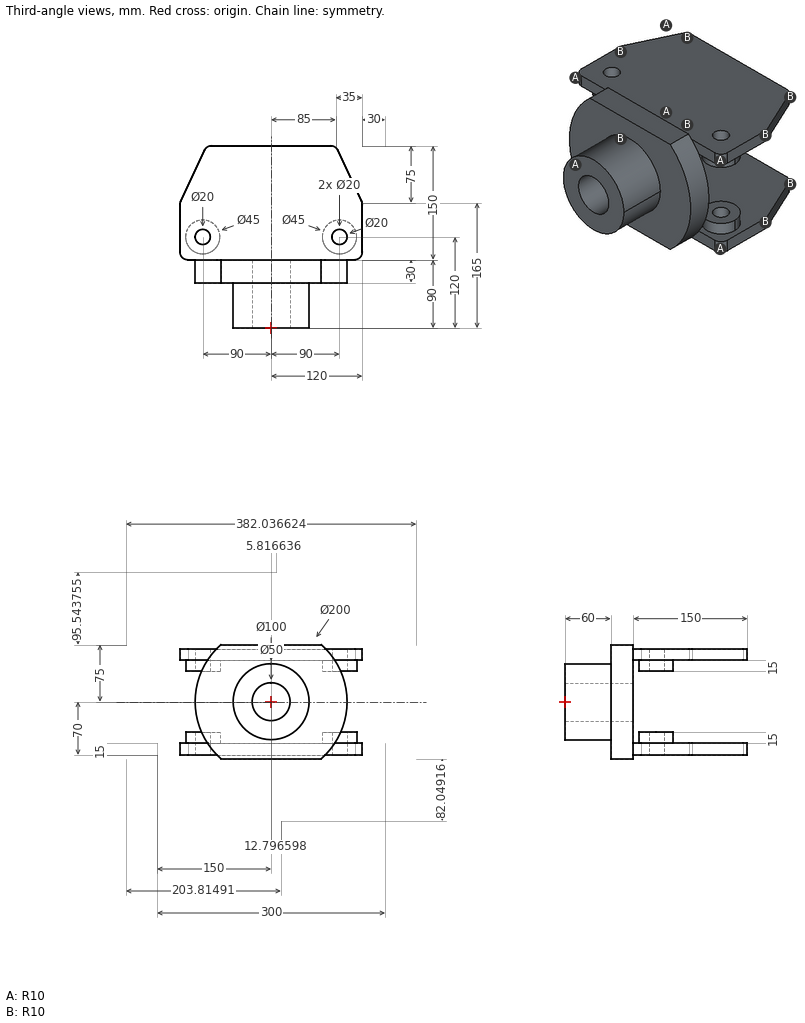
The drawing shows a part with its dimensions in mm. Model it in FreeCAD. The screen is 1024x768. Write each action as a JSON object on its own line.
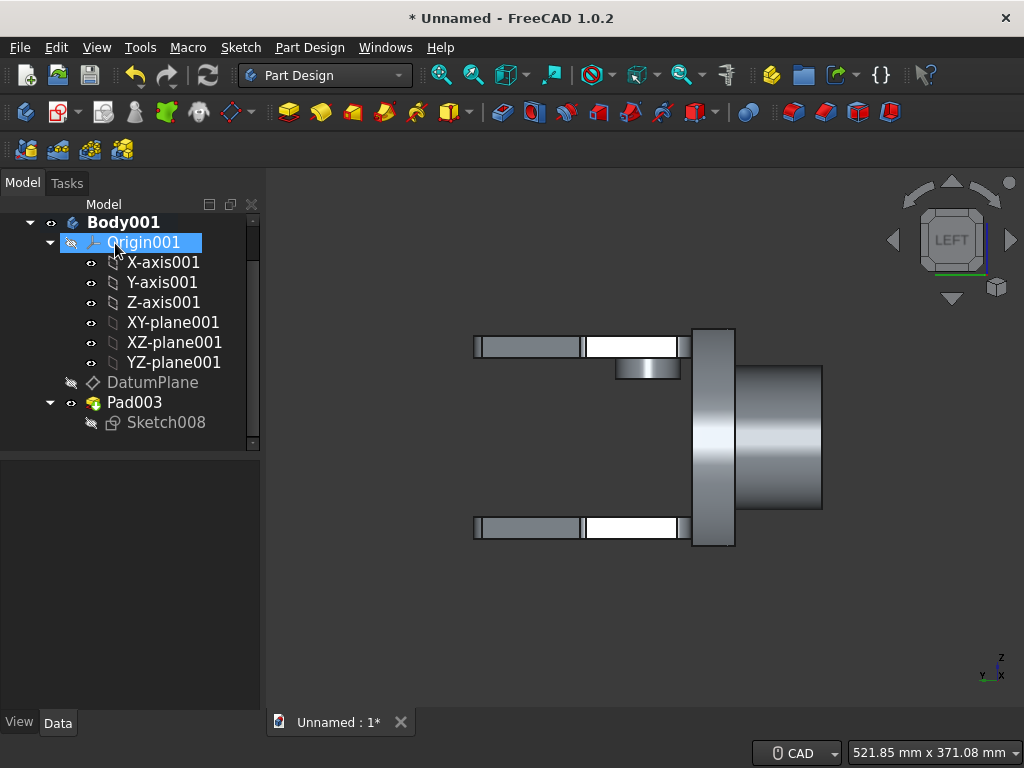
{"action": "left_click", "coordinate": [442, 76]}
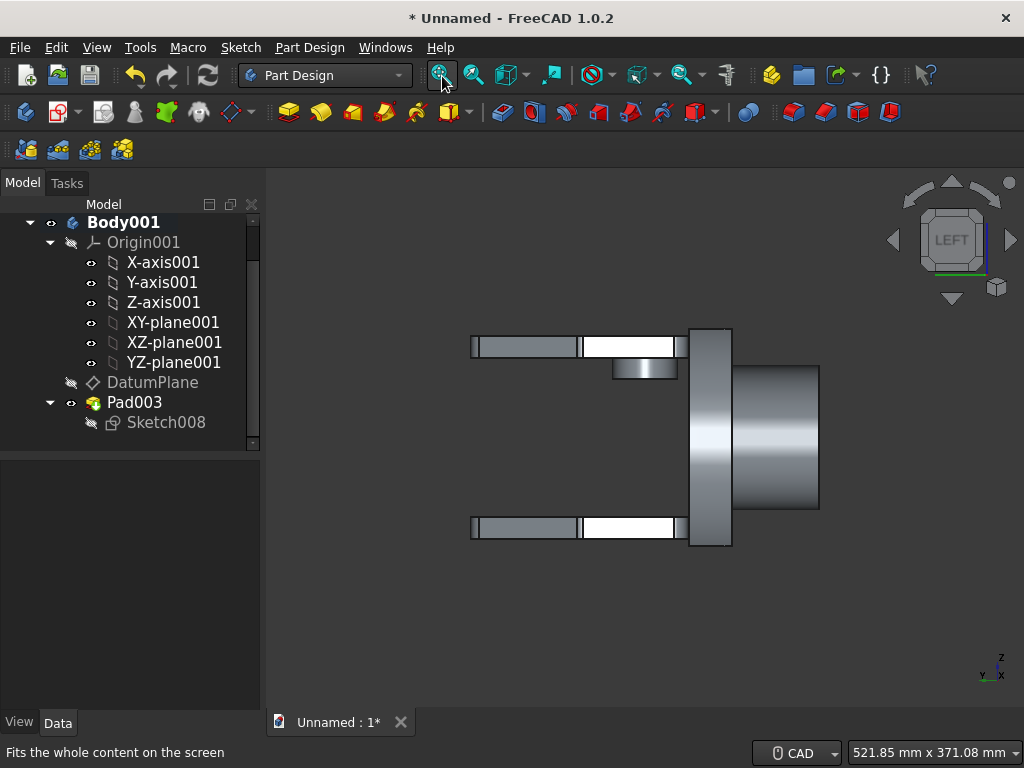
{"action": "left_click", "coordinate": [26, 112]}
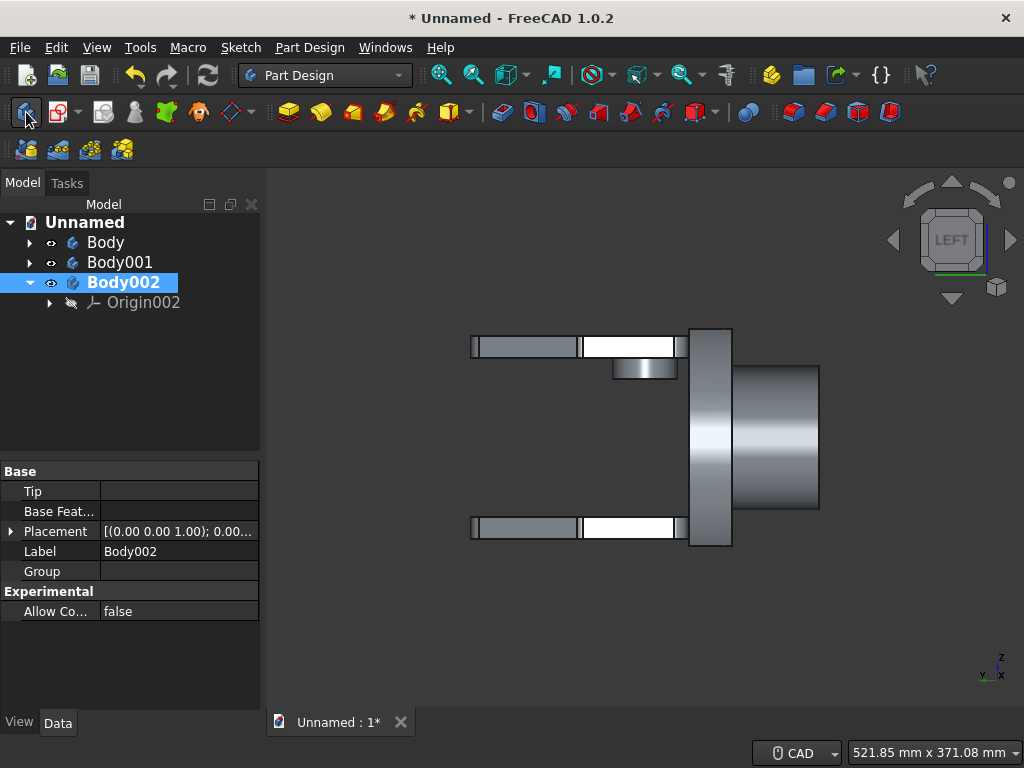
{"action": "left_click", "coordinate": [50, 303]}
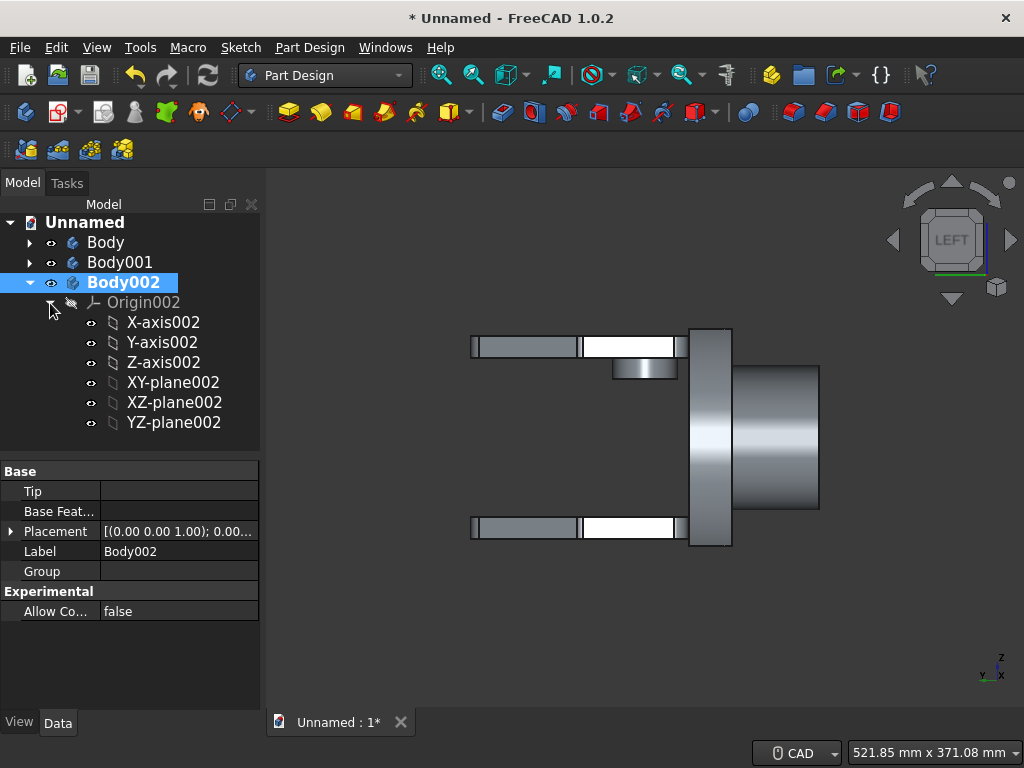
{"action": "left_click", "coordinate": [136, 383]}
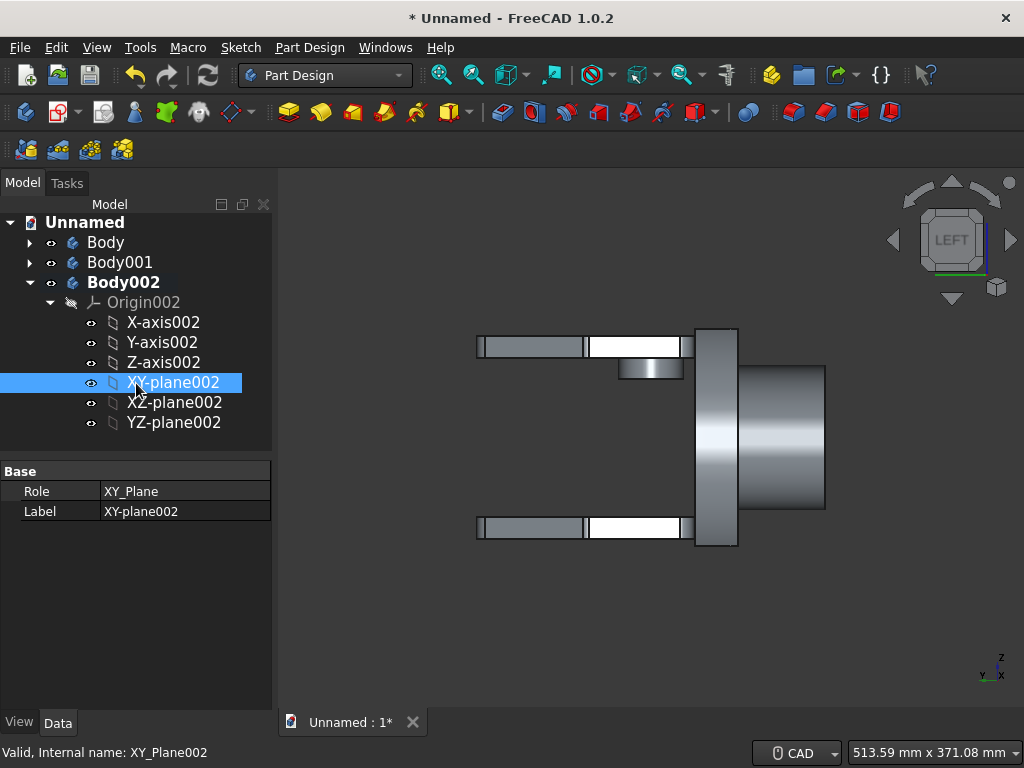
{"action": "left_click", "coordinate": [232, 112]}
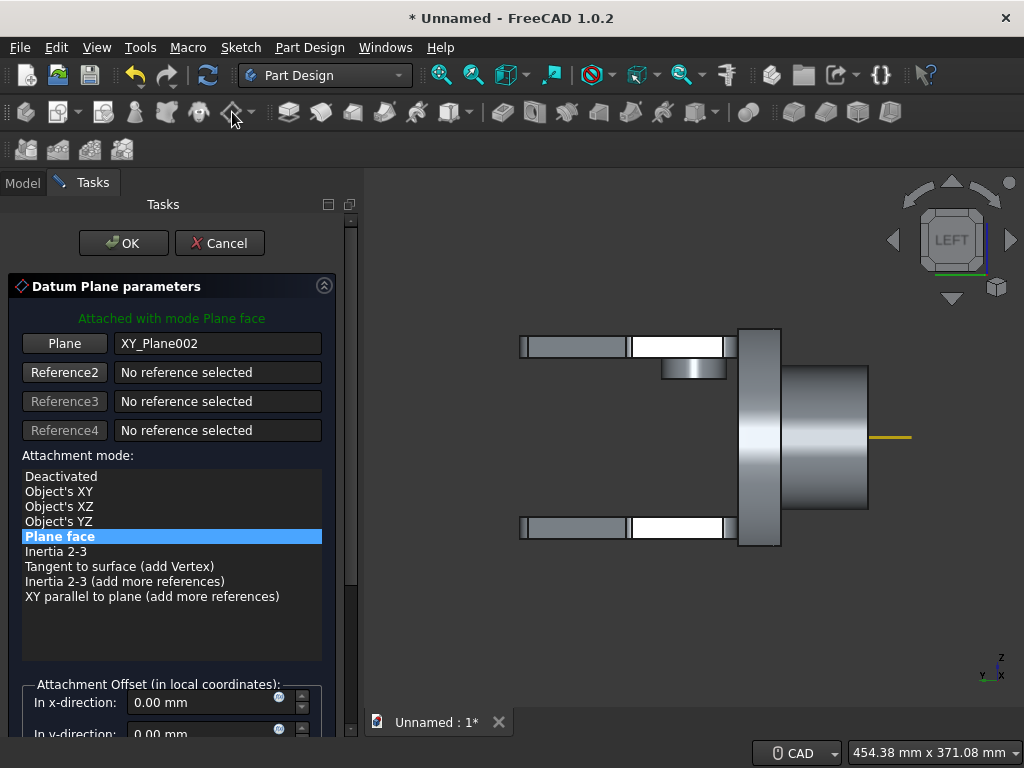
{"action": "scroll", "coordinate": [351, 475], "scroll_direction": "down", "scroll_amount": 2}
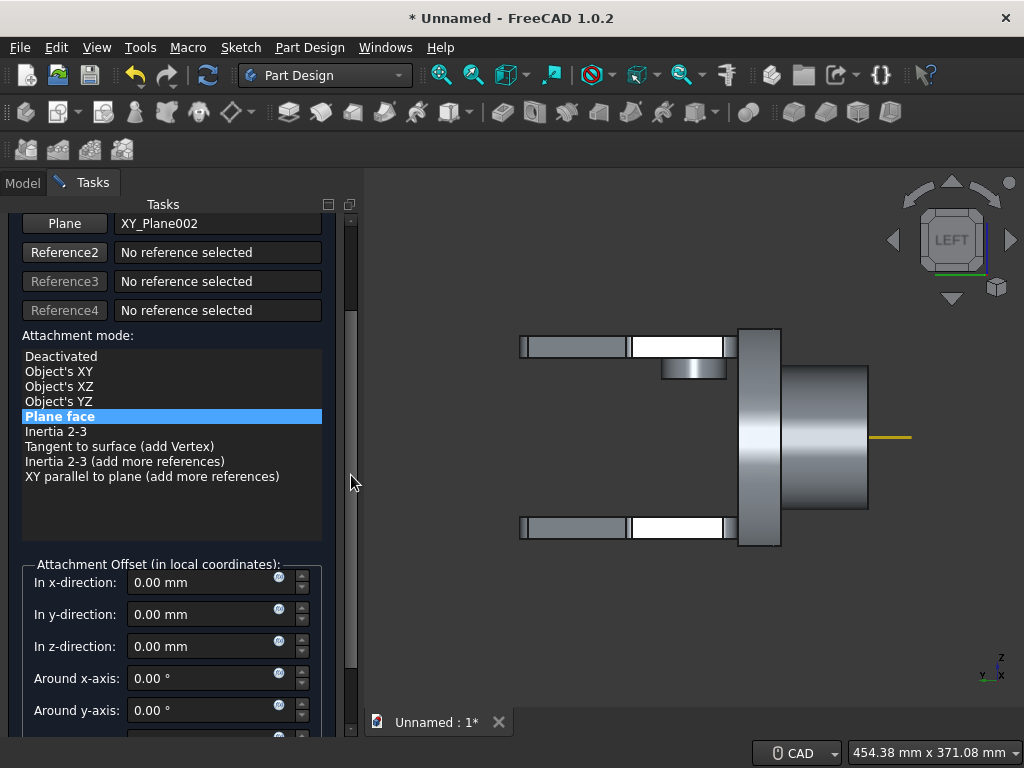
{"action": "triple_click", "coordinate": [210, 646]}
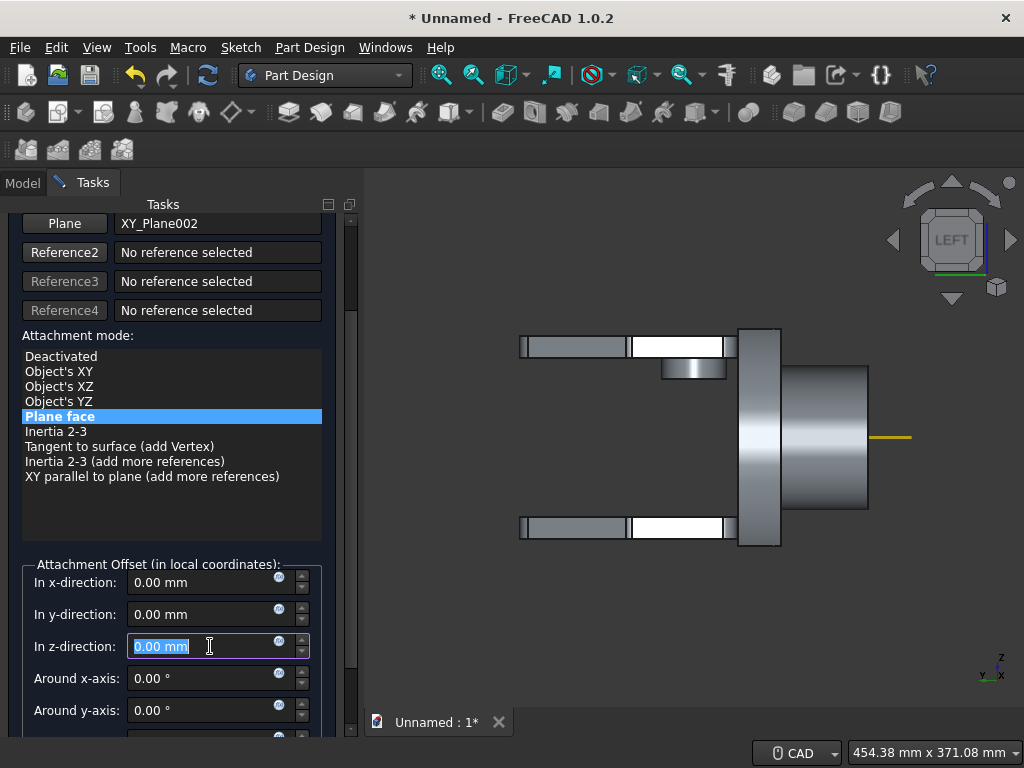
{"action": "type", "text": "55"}
{"action": "key", "text": "Tab"}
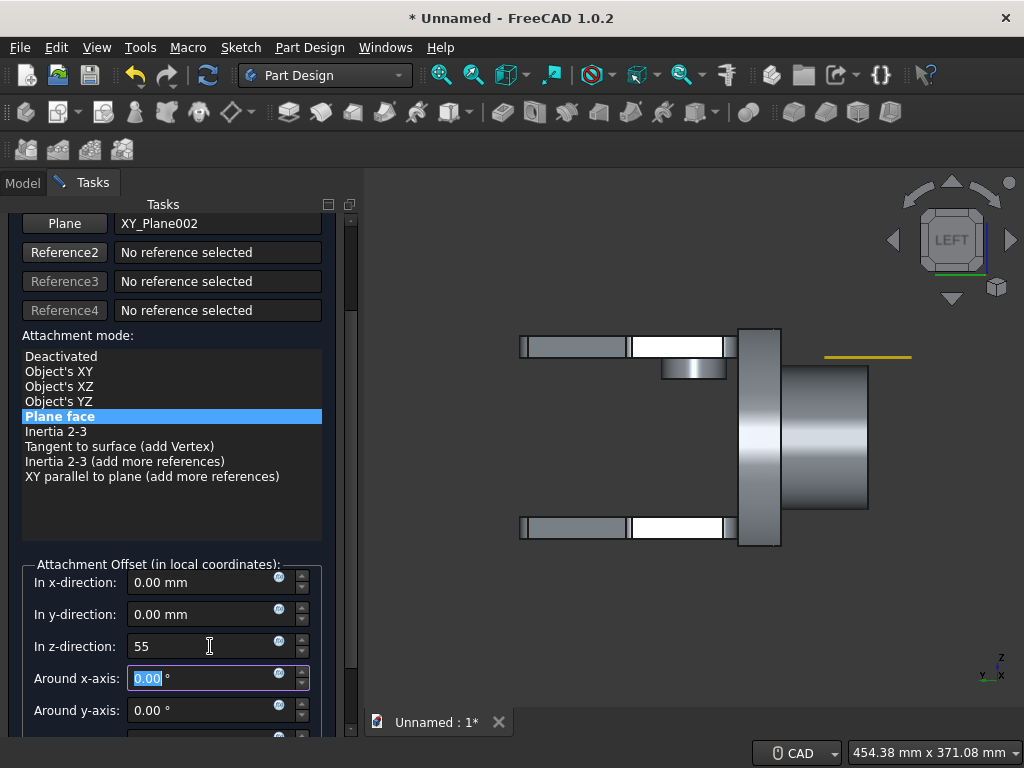
{"action": "scroll", "coordinate": [351, 475], "scroll_direction": "up", "scroll_amount": 3}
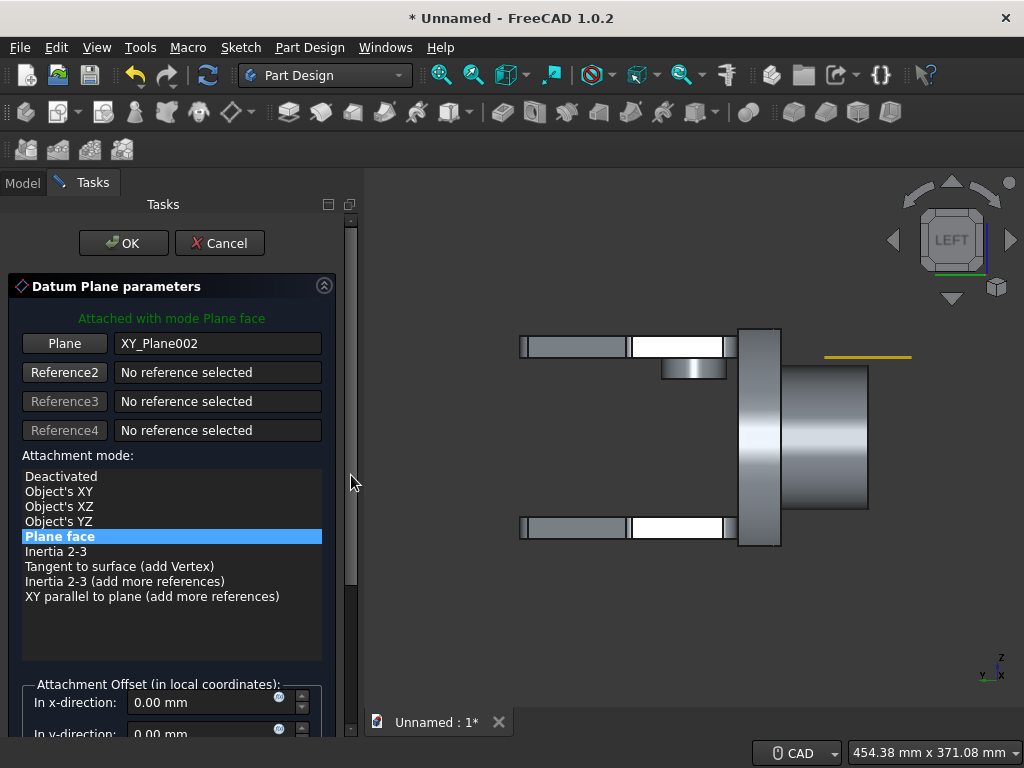
{"action": "left_click", "coordinate": [124, 243]}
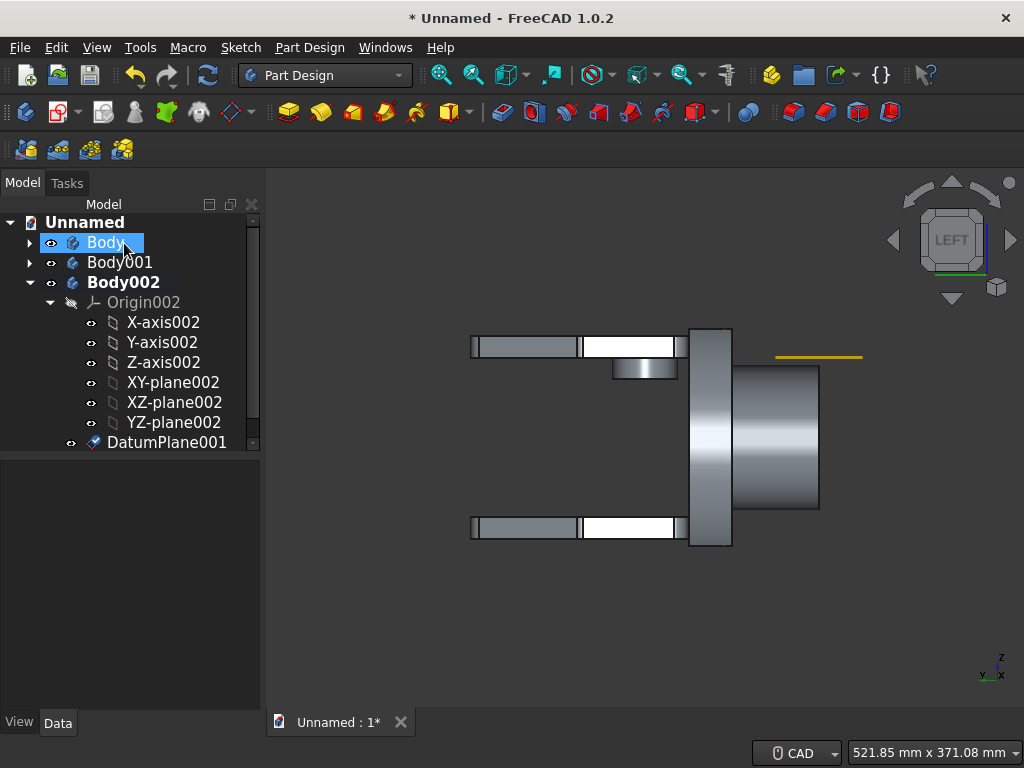
{"action": "left_click", "coordinate": [116, 443]}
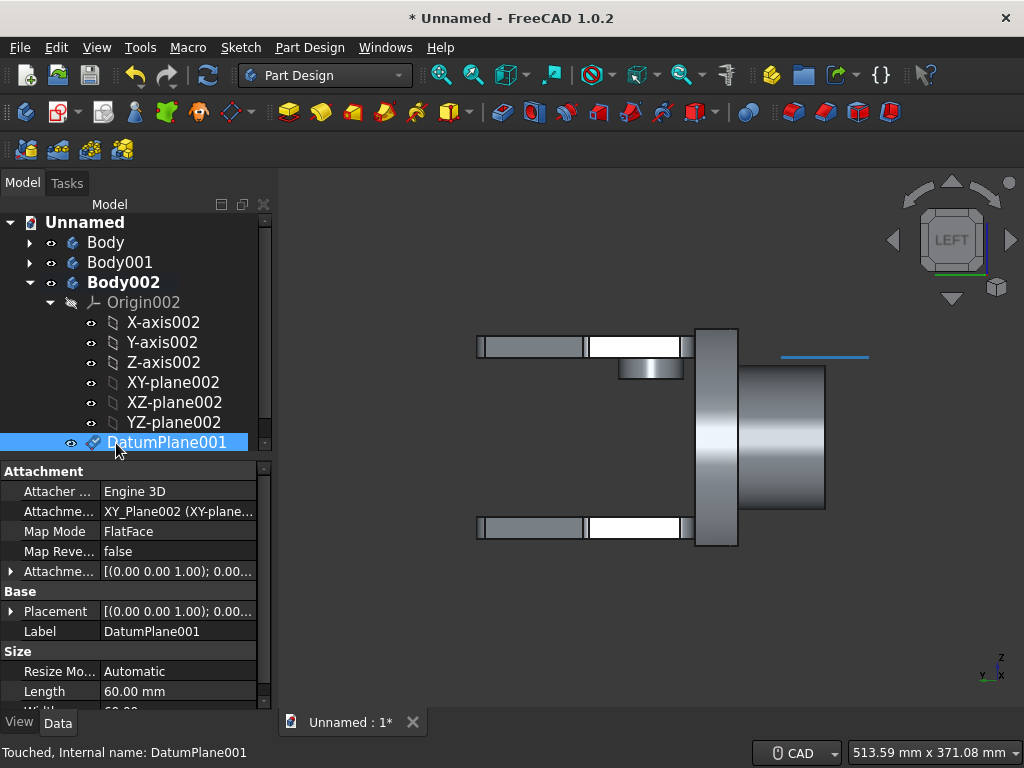
{"action": "left_click", "coordinate": [58, 112]}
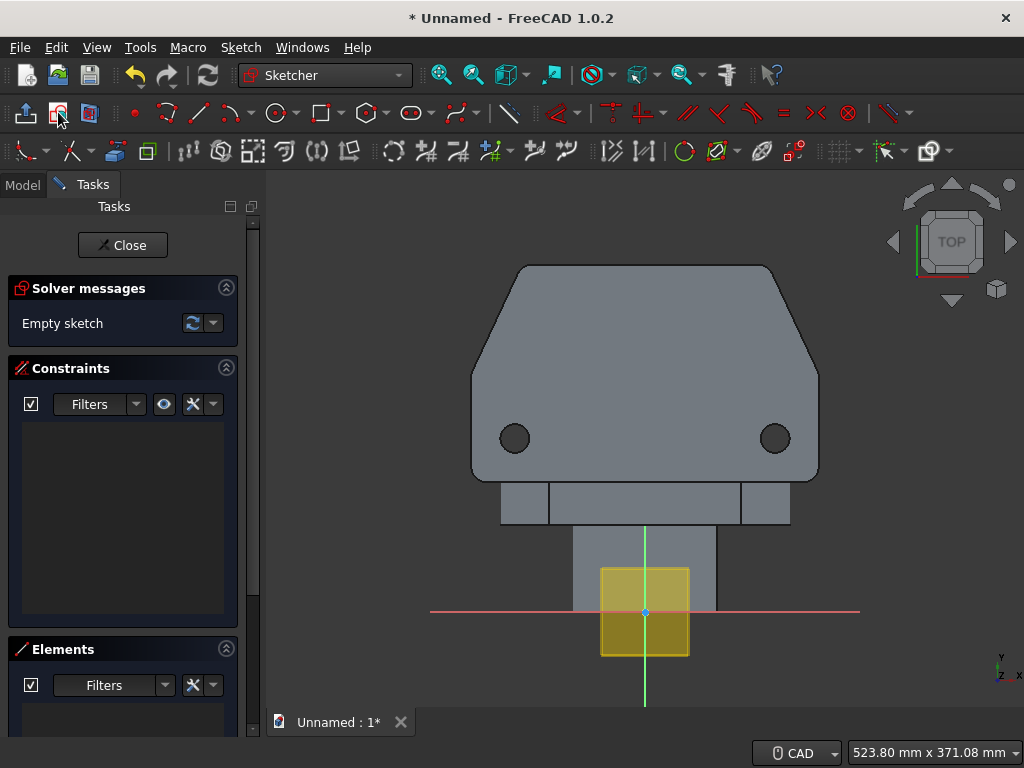
{"action": "scroll", "coordinate": [826, 439], "scroll_direction": "up", "scroll_amount": 8}